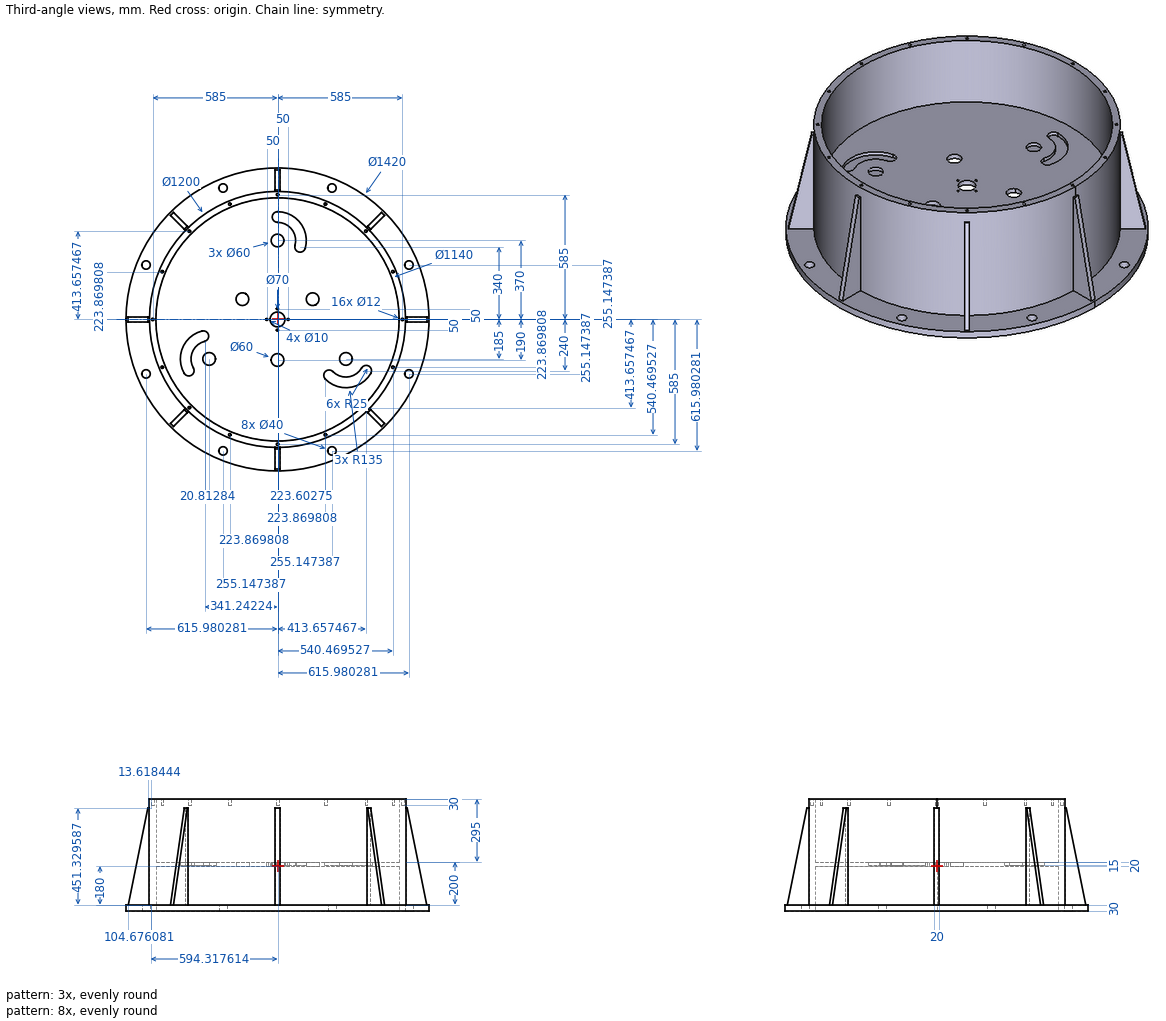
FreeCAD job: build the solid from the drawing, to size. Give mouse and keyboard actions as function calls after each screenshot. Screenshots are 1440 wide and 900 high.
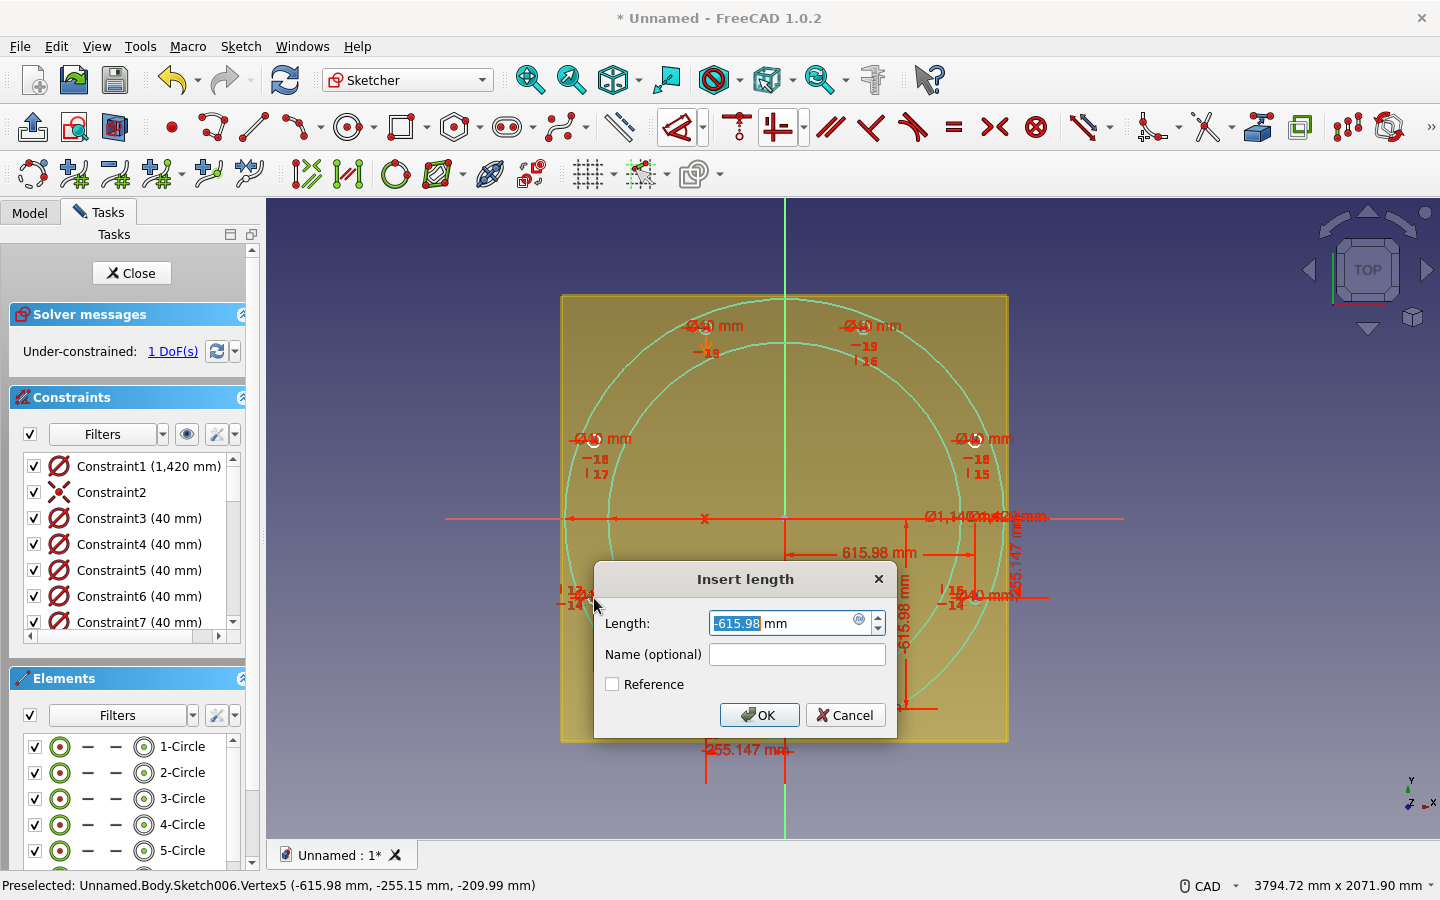
text(-615.980281)
key(Return)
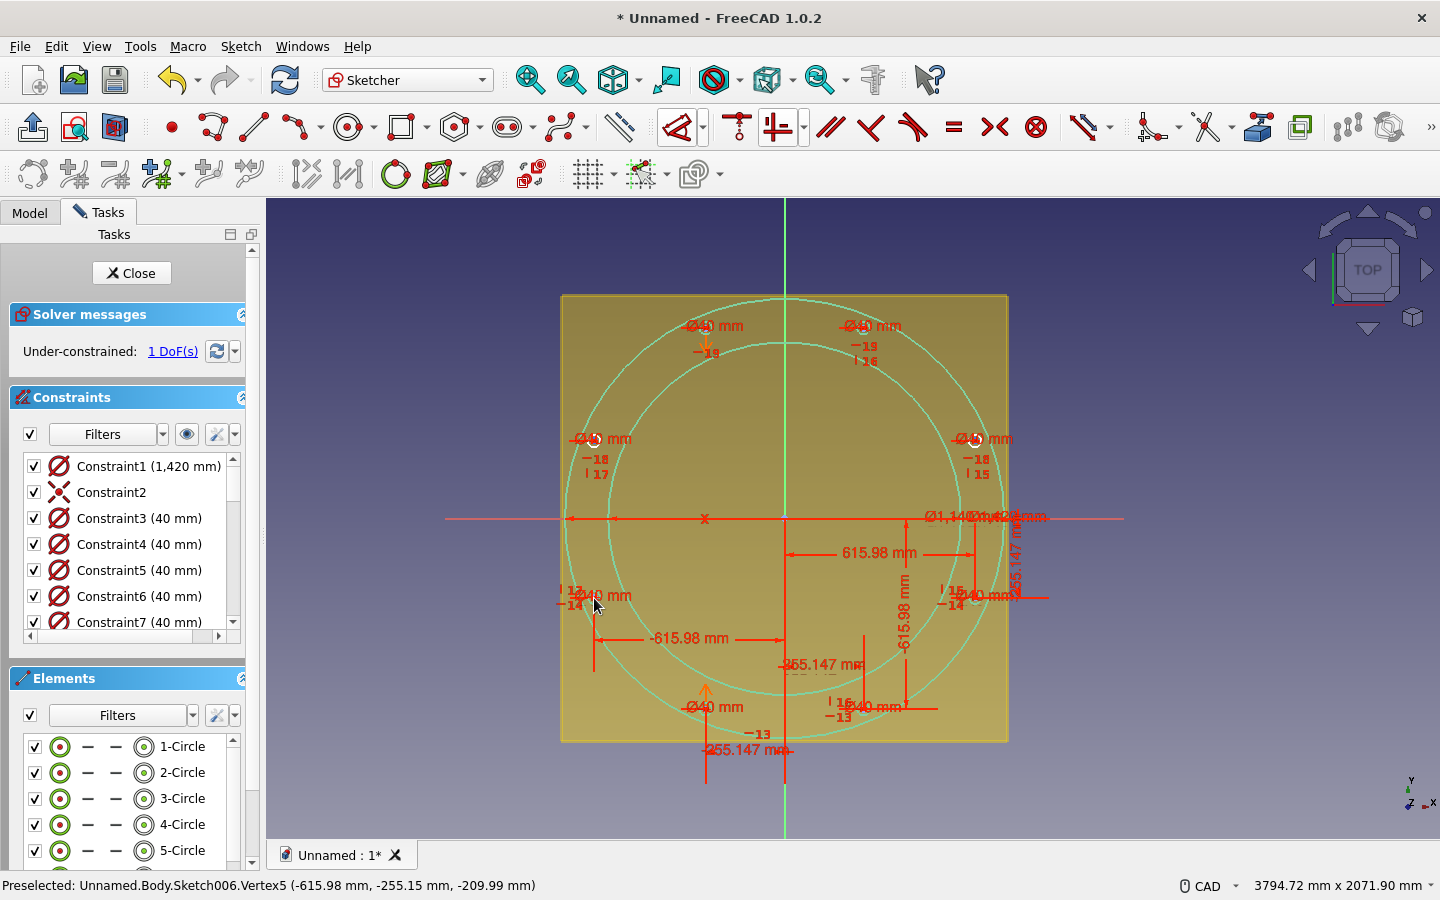
click(975, 441)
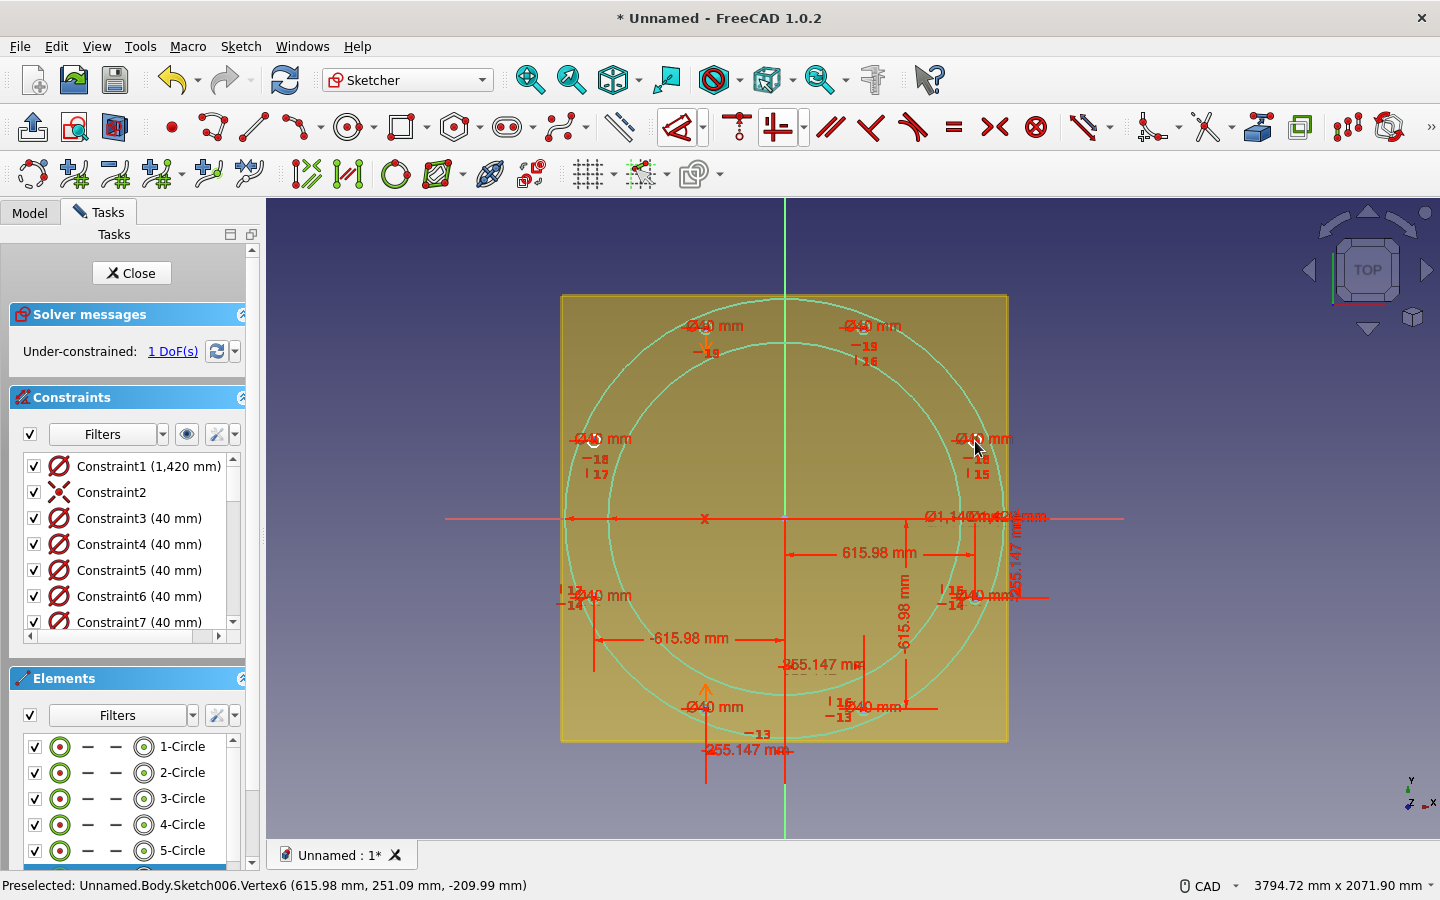
key(i)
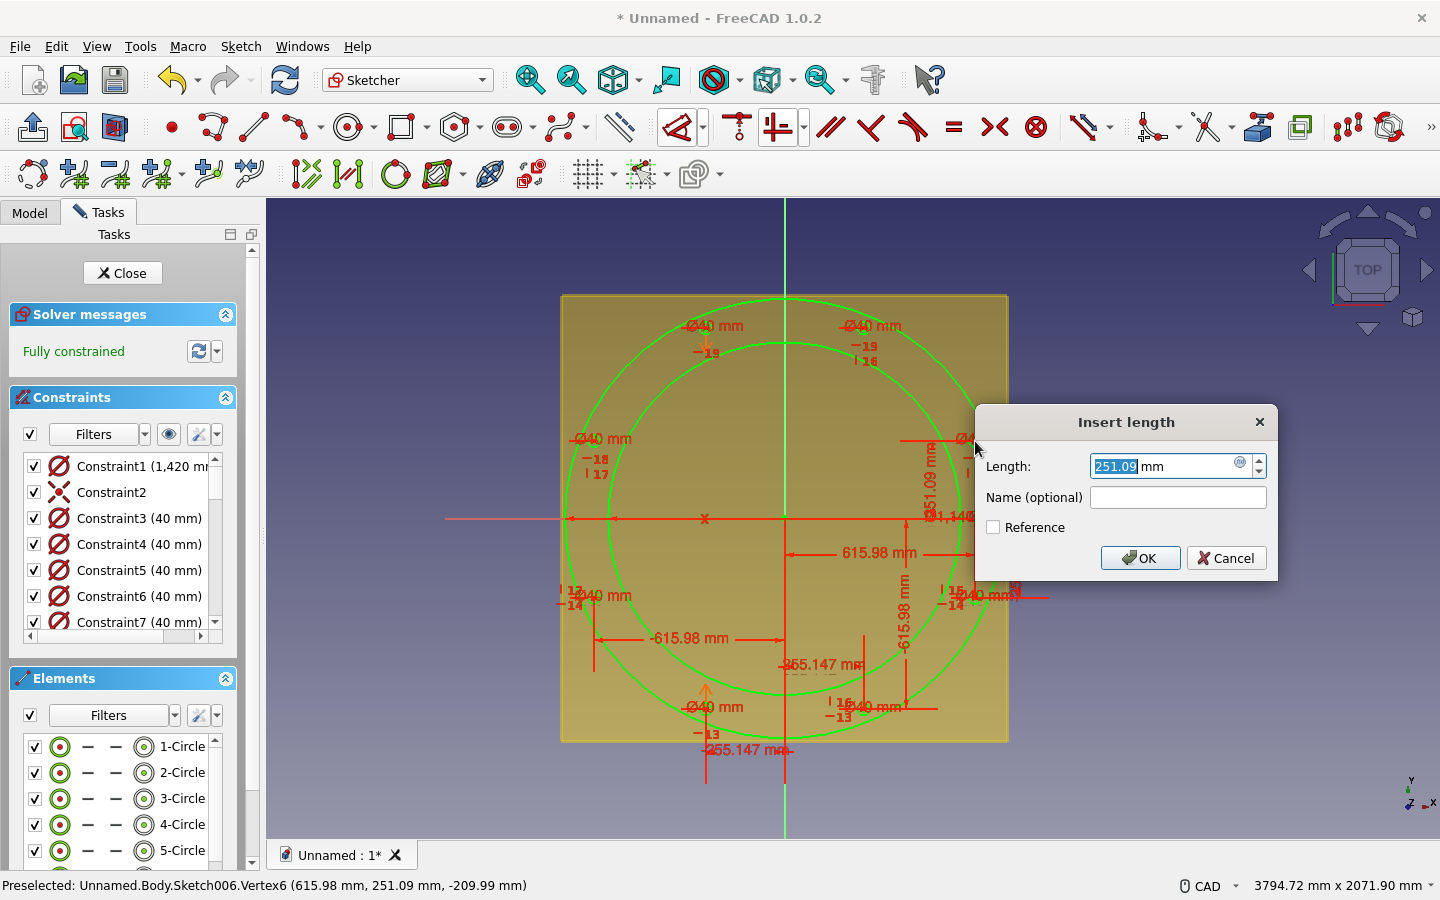
text(255.147387)
key(Return)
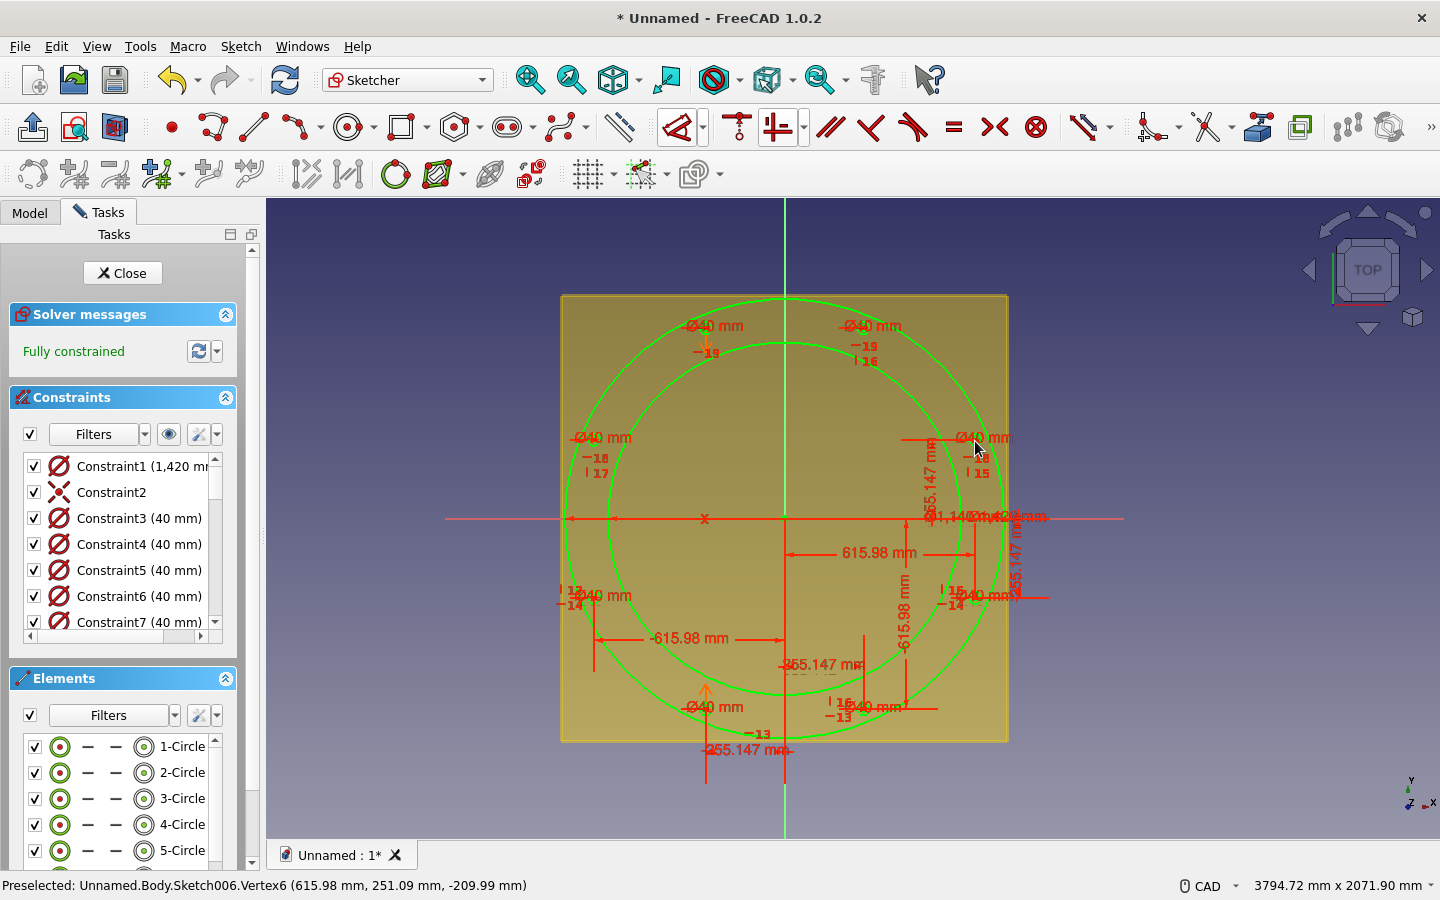
click(123, 273)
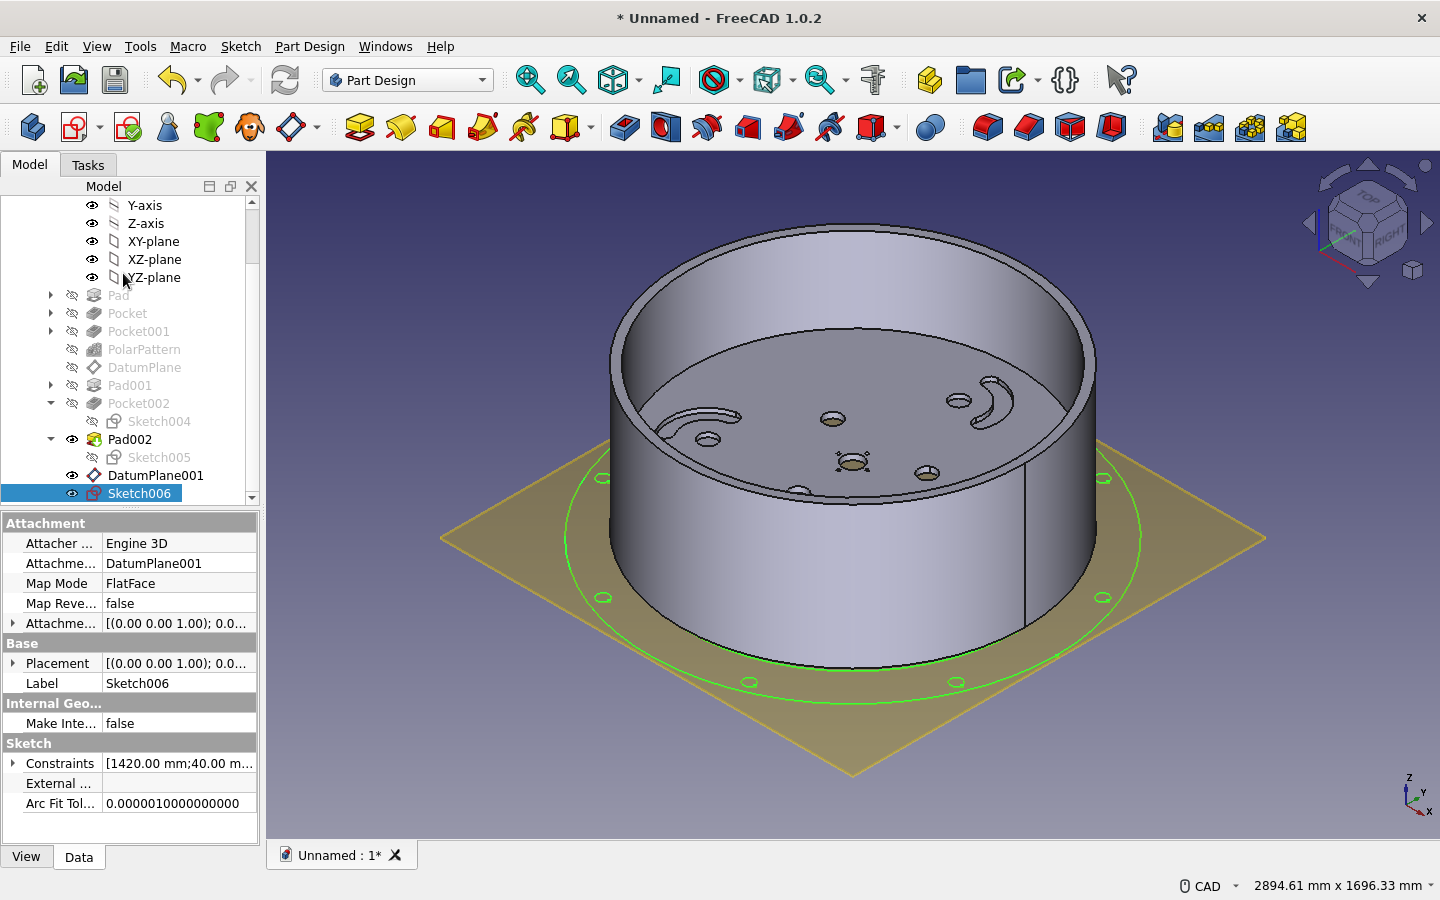
click(360, 128)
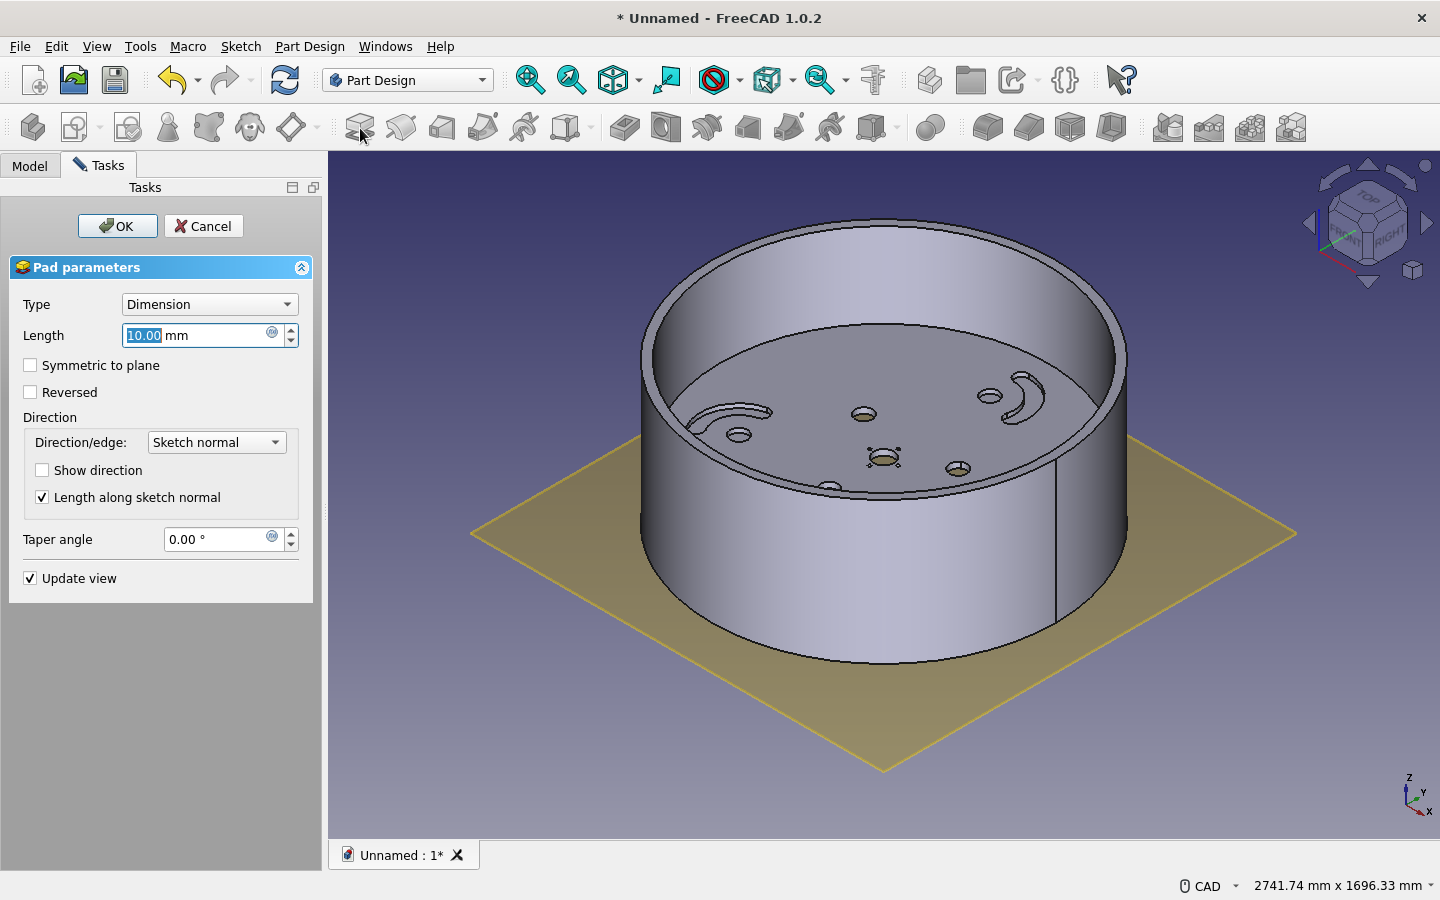
text(30)
key(Tab)